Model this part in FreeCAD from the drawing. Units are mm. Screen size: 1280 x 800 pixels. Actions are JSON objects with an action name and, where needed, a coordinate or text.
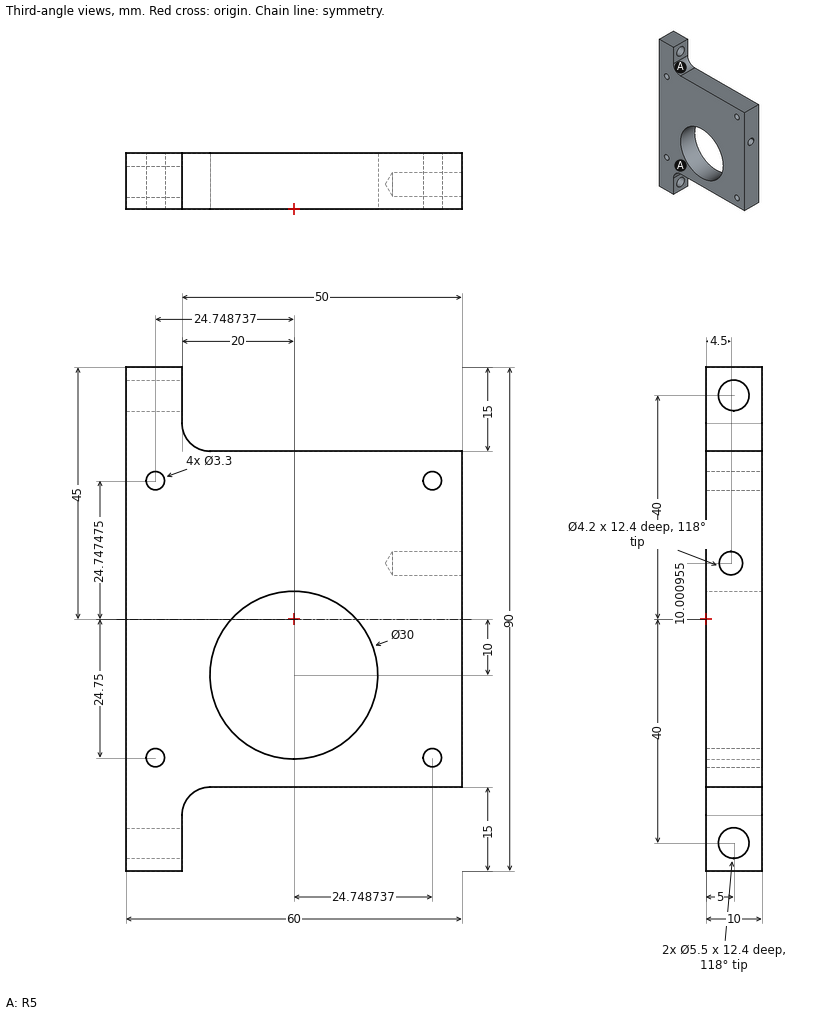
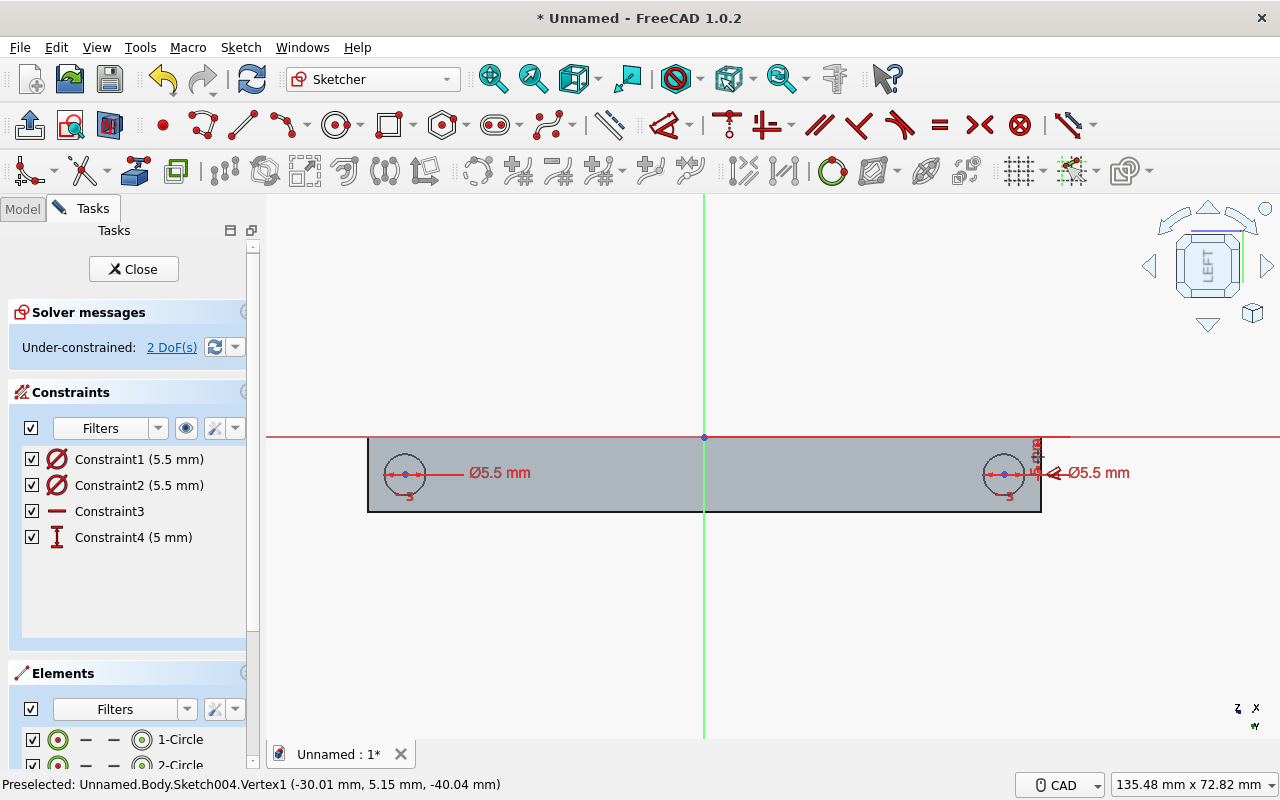
{"action": "left_click", "coordinate": [1004, 475]}
{"action": "left_click", "coordinate": [854, 403]}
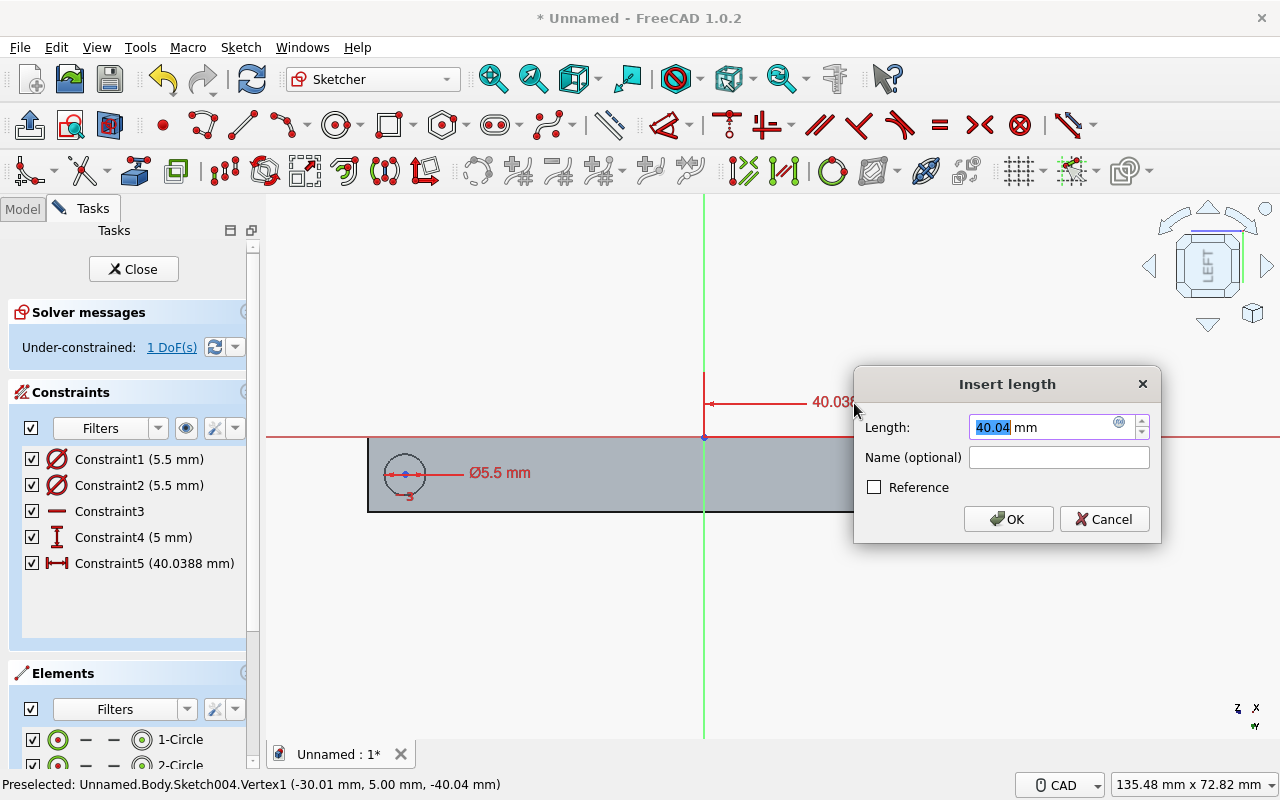
{"action": "type", "text": "40"}
{"action": "key", "text": "Return"}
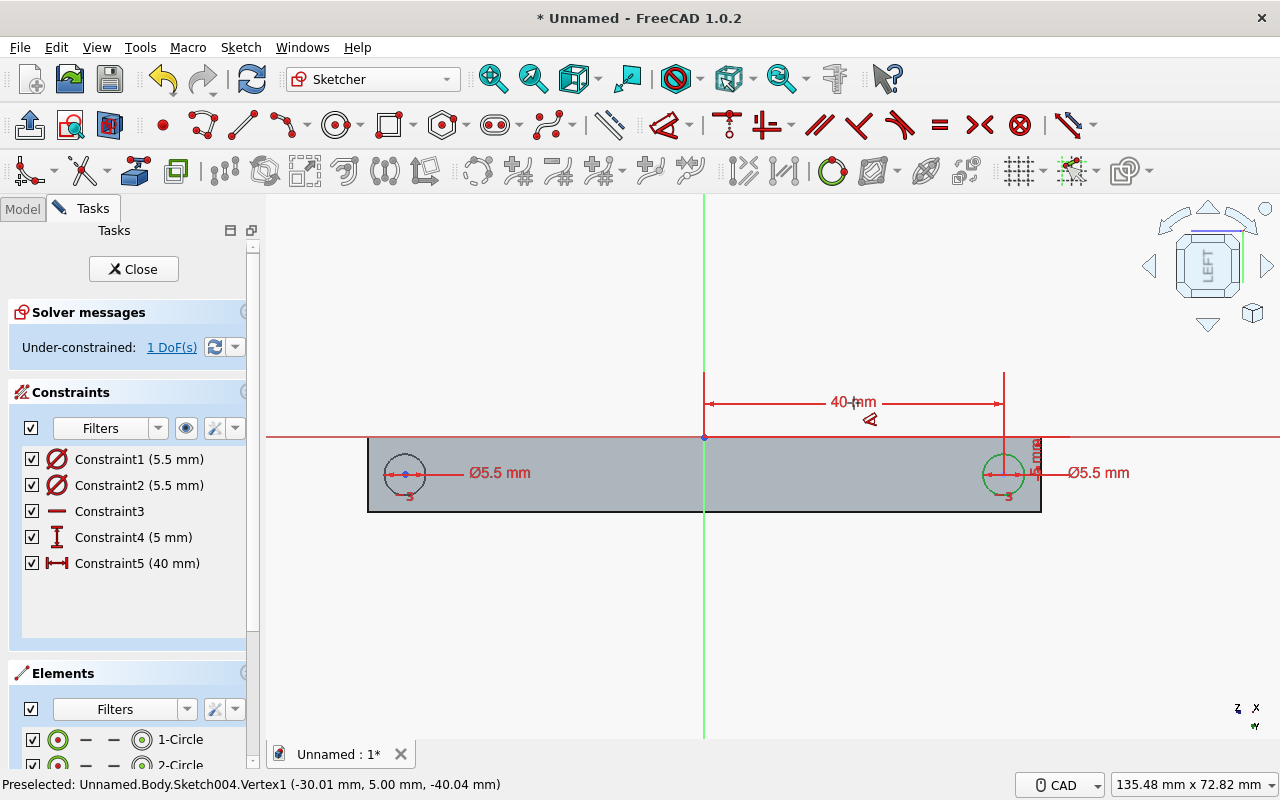
{"action": "left_click", "coordinate": [405, 475]}
{"action": "left_click", "coordinate": [555, 403]}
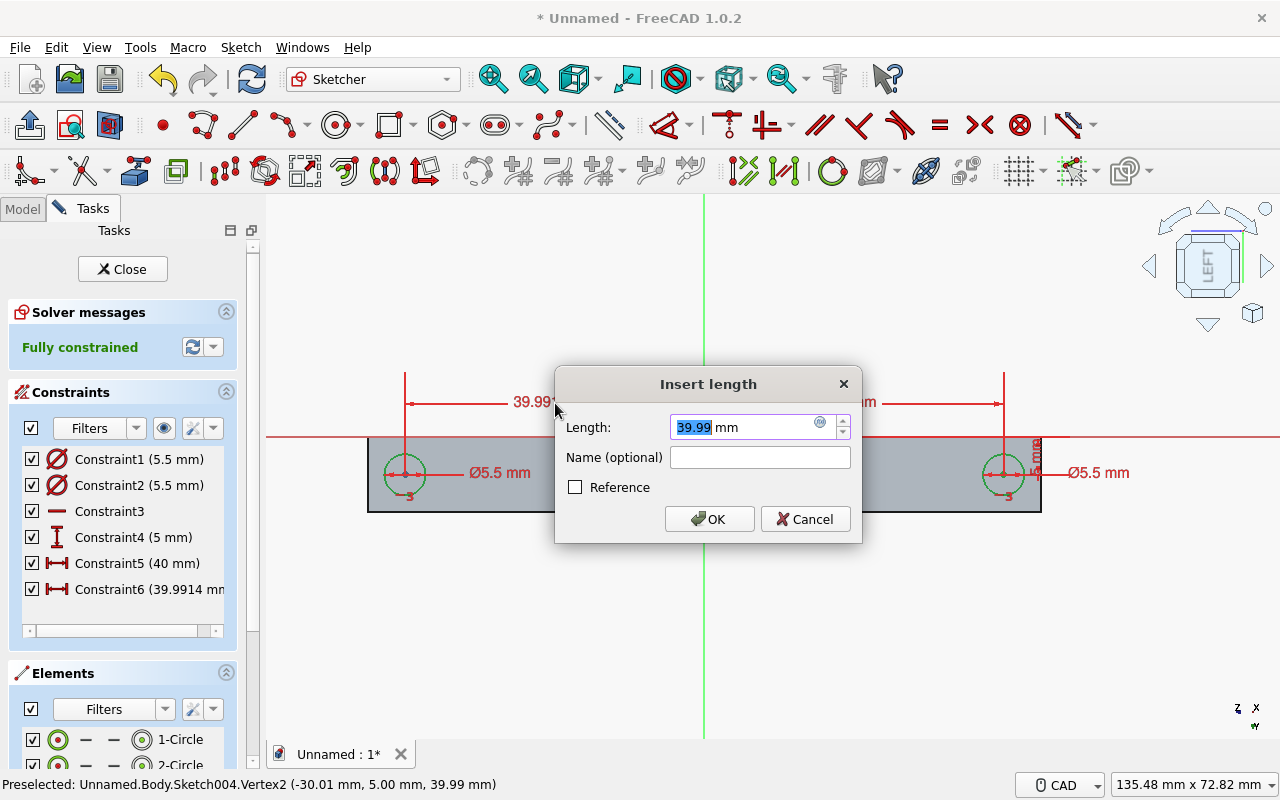
{"action": "type", "text": "40"}
{"action": "key", "text": "Return"}
{"action": "key", "text": "Escape"}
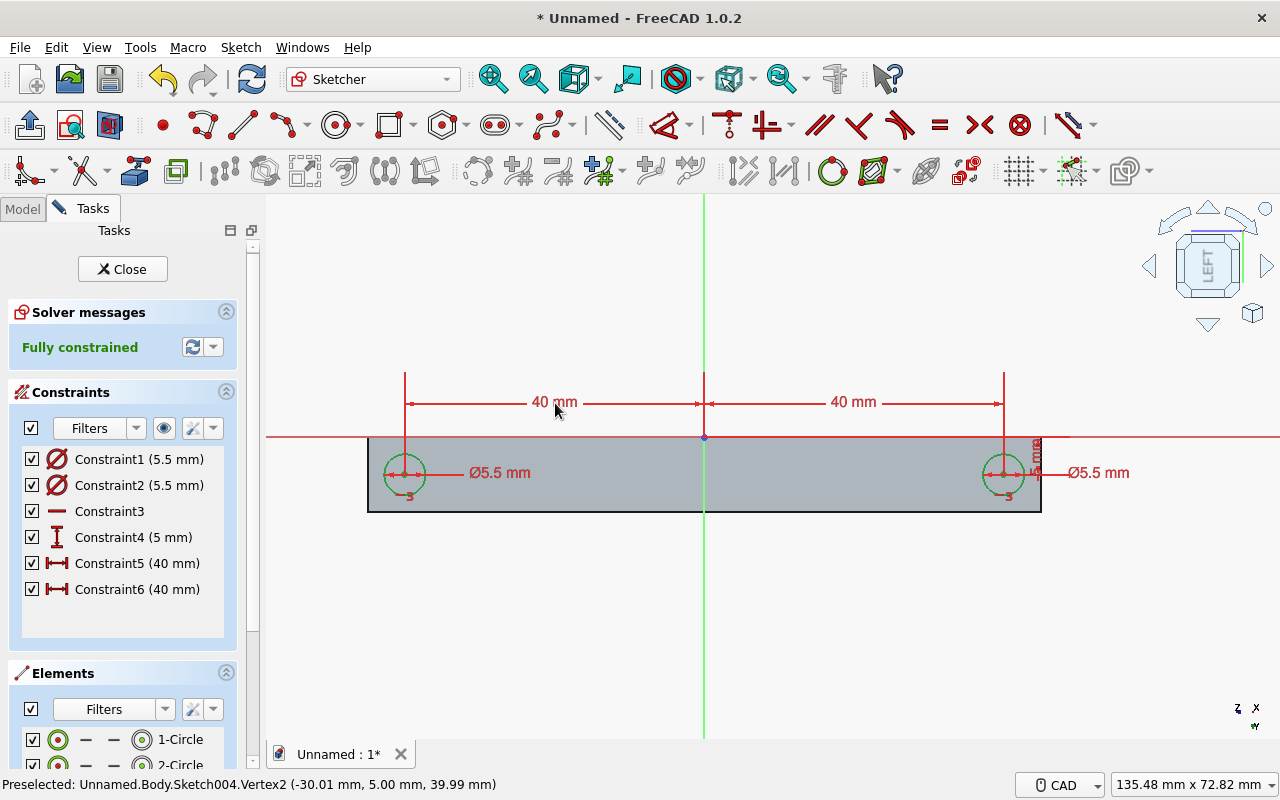
{"action": "left_click", "coordinate": [123, 269]}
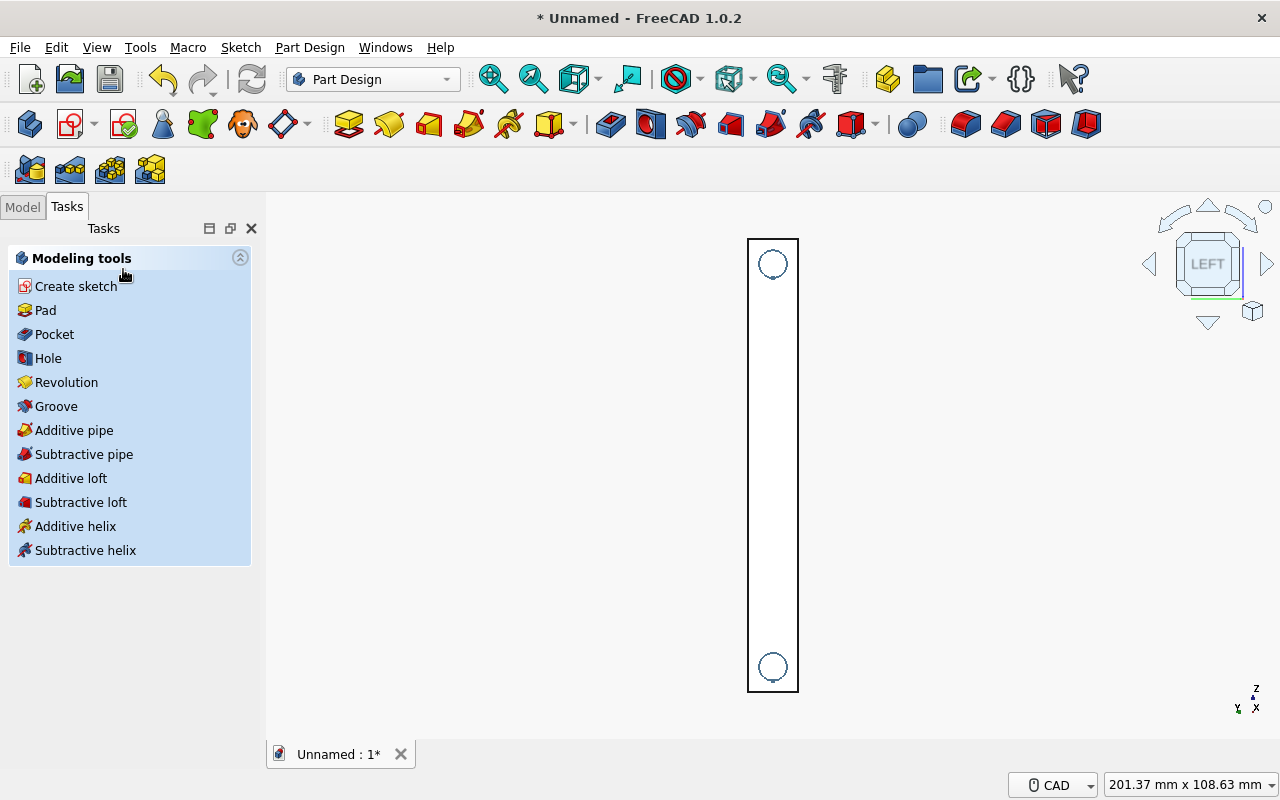
{"action": "left_click", "coordinate": [652, 124]}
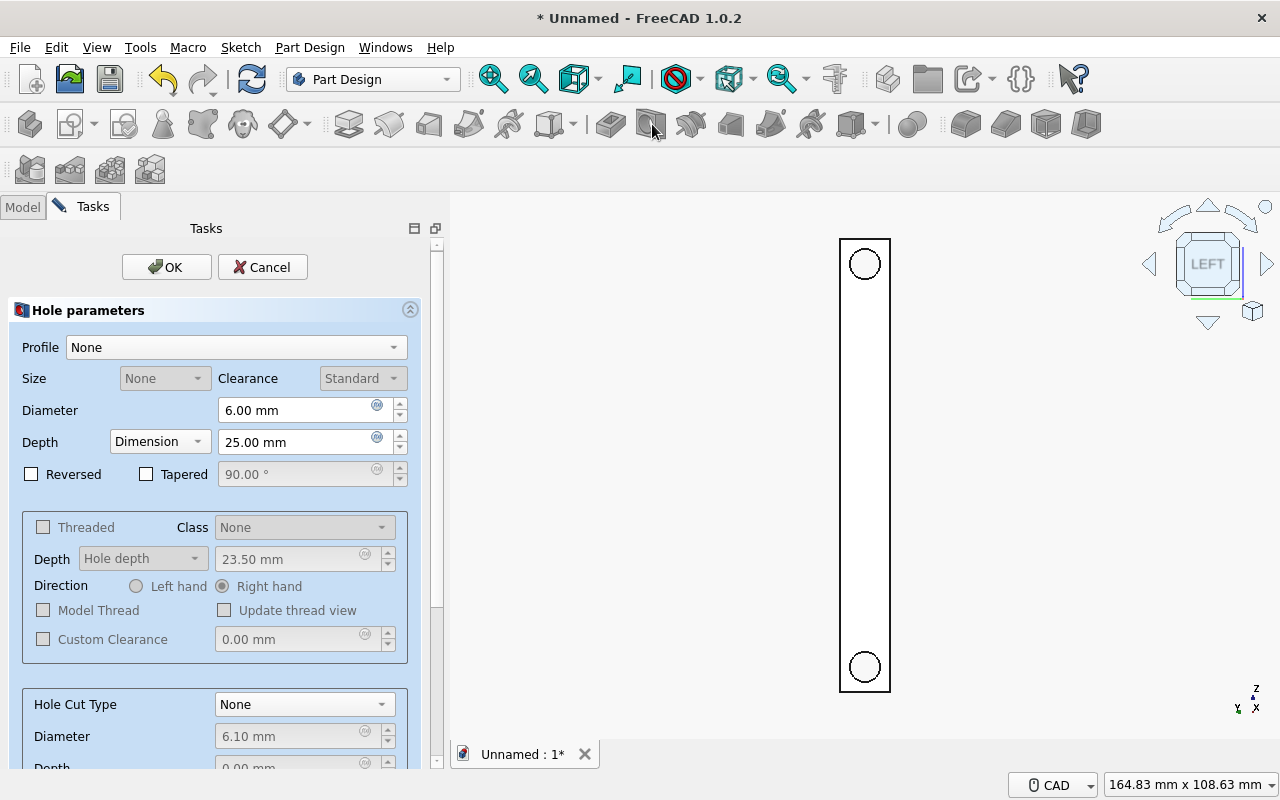
{"action": "triple_click", "coordinate": [305, 410]}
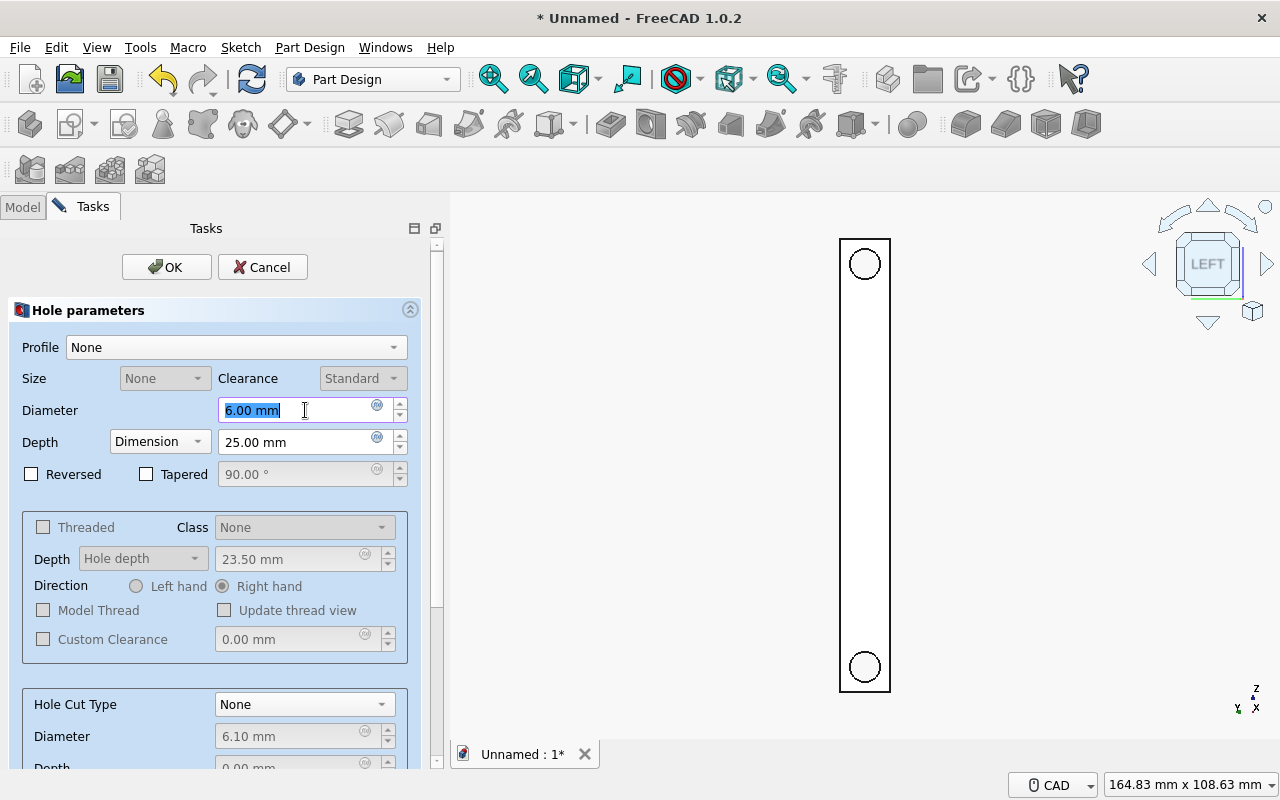
{"action": "type", "text": "5.5"}
{"action": "key", "text": "Tab"}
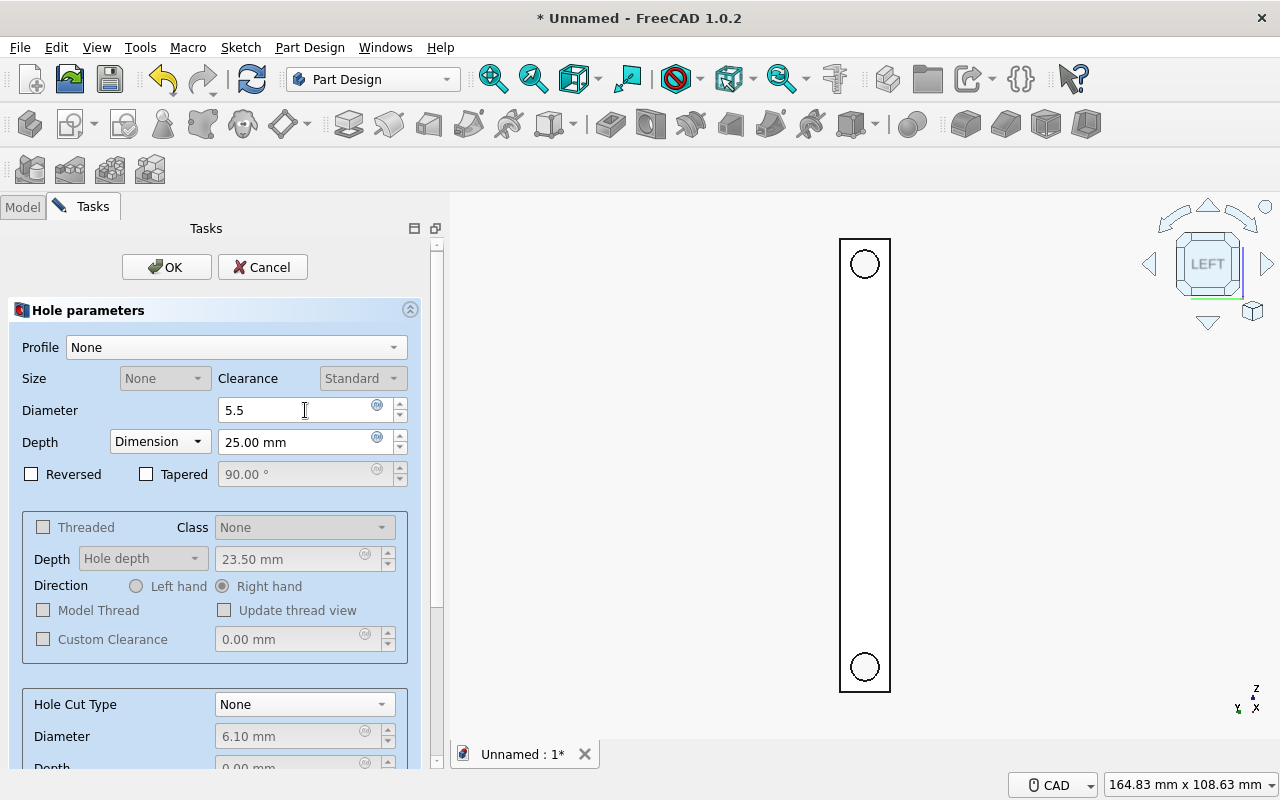
{"action": "triple_click", "coordinate": [305, 442]}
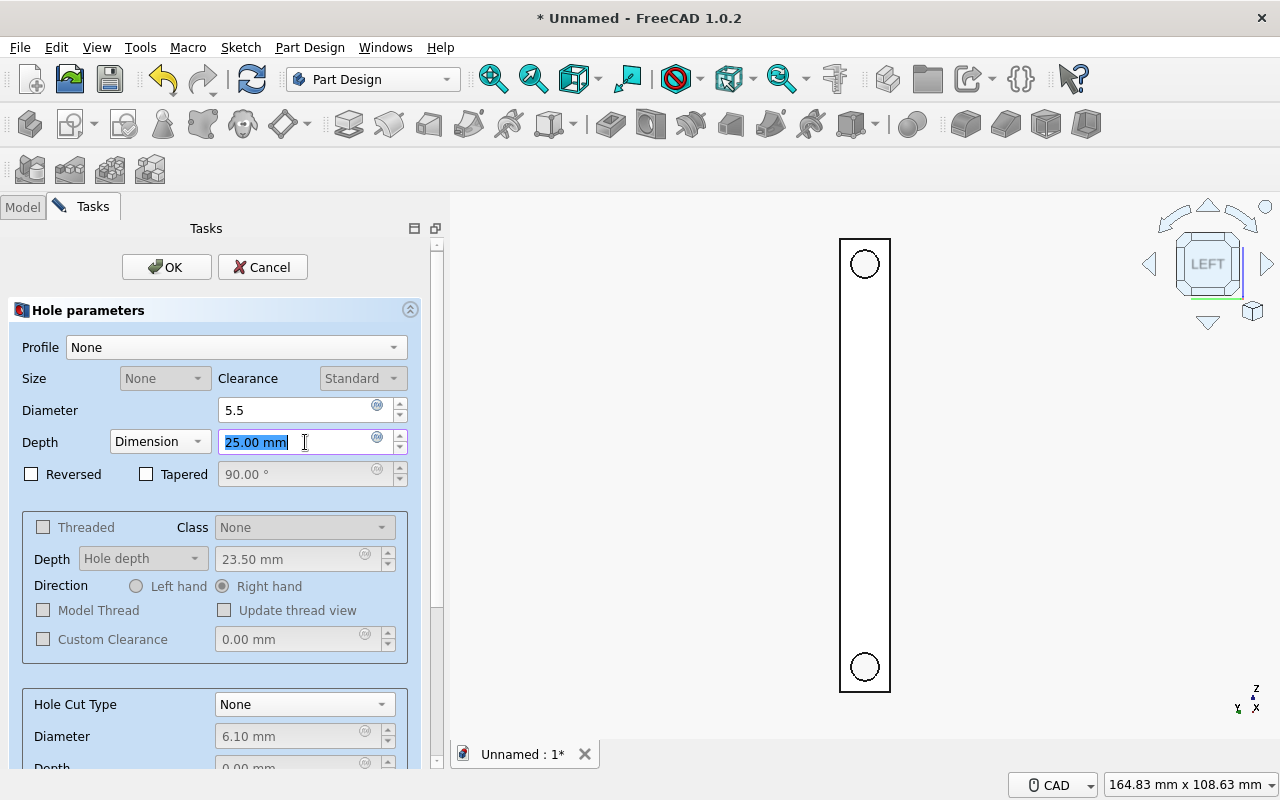
{"action": "type", "text": "12.4"}
{"action": "key", "text": "Tab"}